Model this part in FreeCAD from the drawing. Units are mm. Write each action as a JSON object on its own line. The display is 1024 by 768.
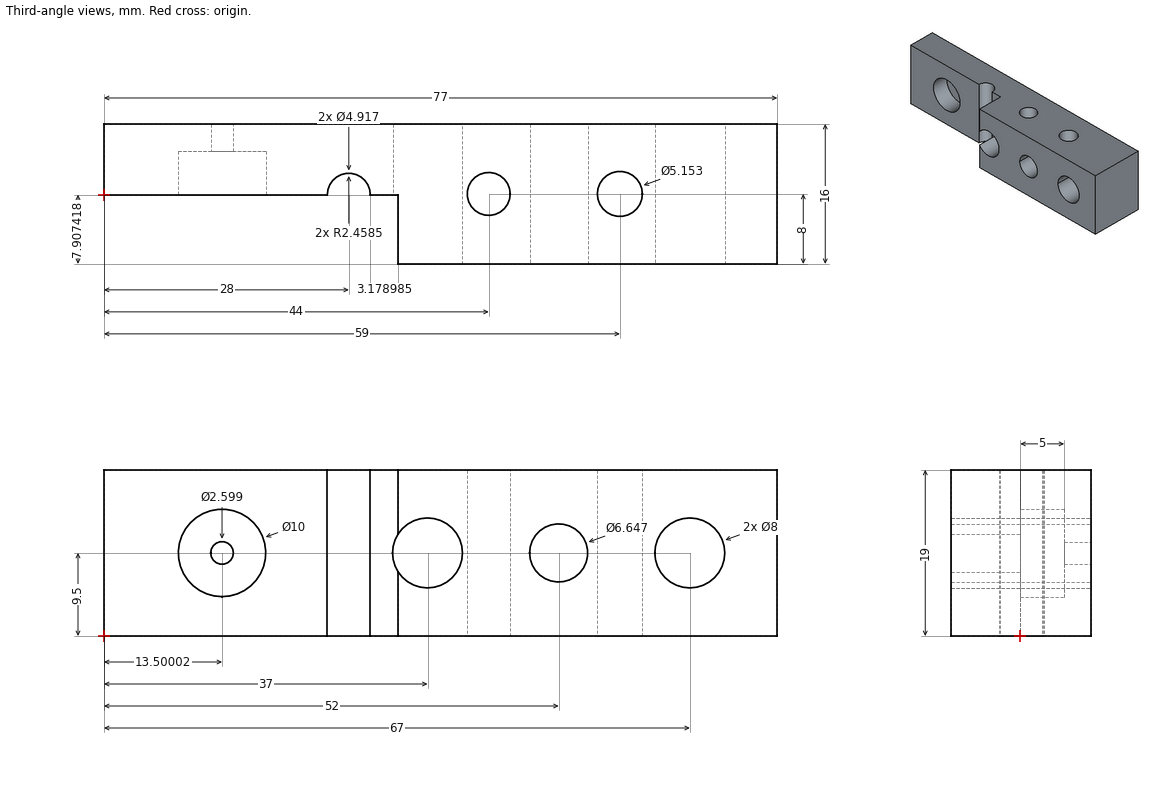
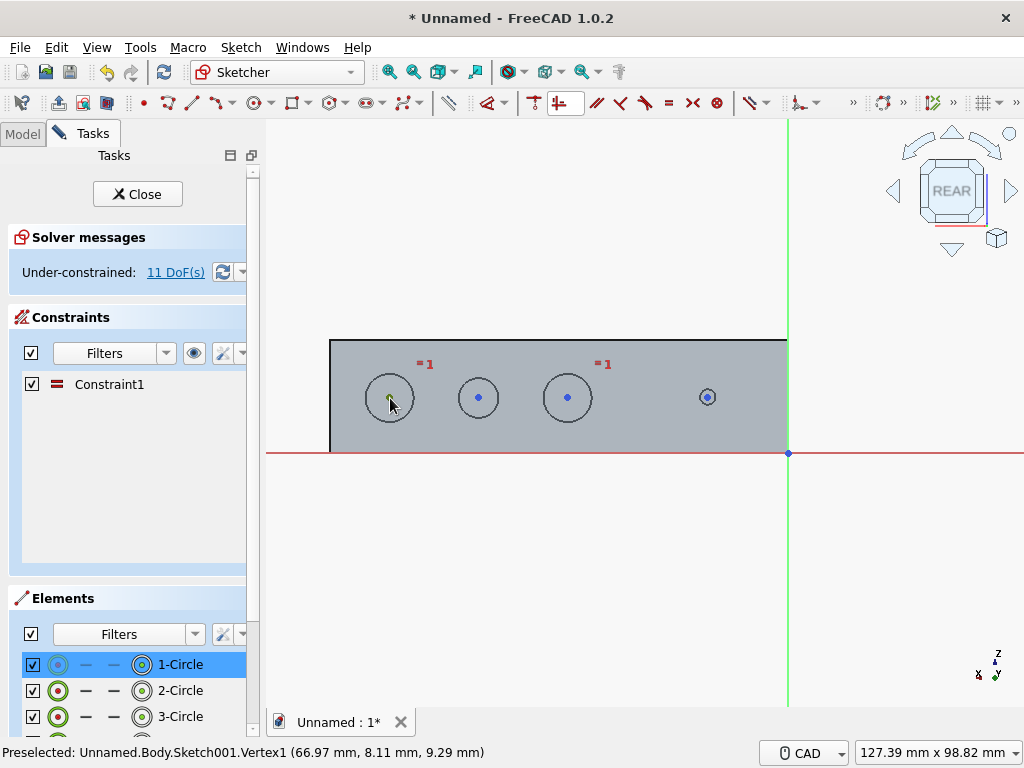
{"action": "left_click", "coordinate": [479, 398]}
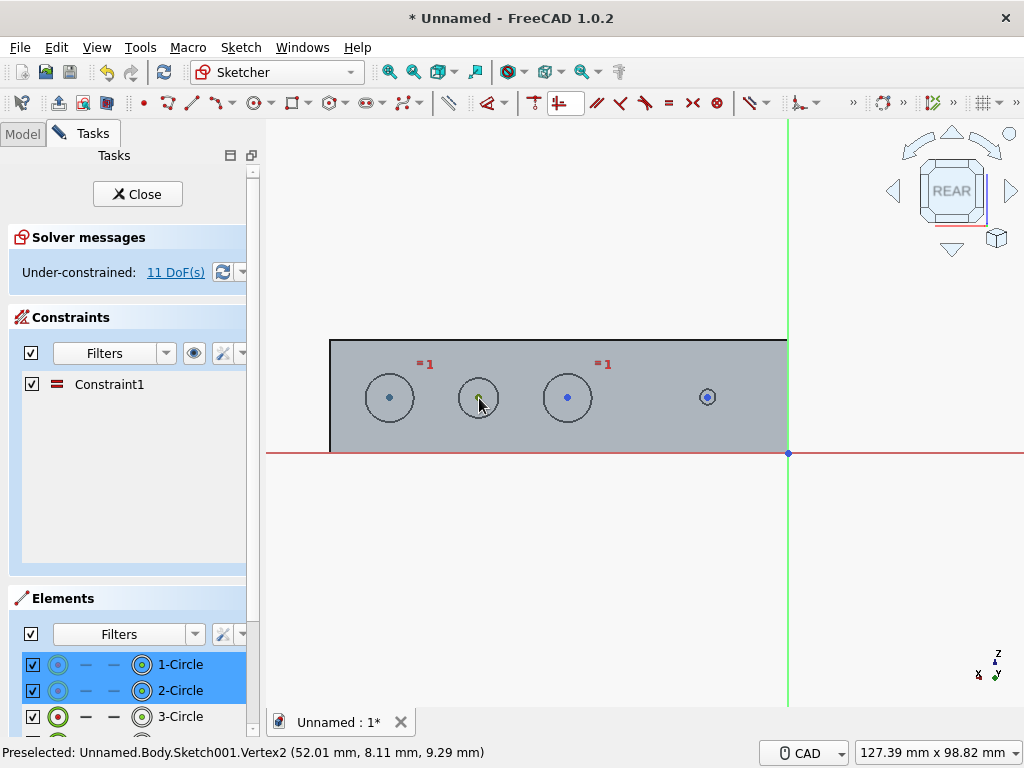
{"action": "left_click", "coordinate": [578, 104]}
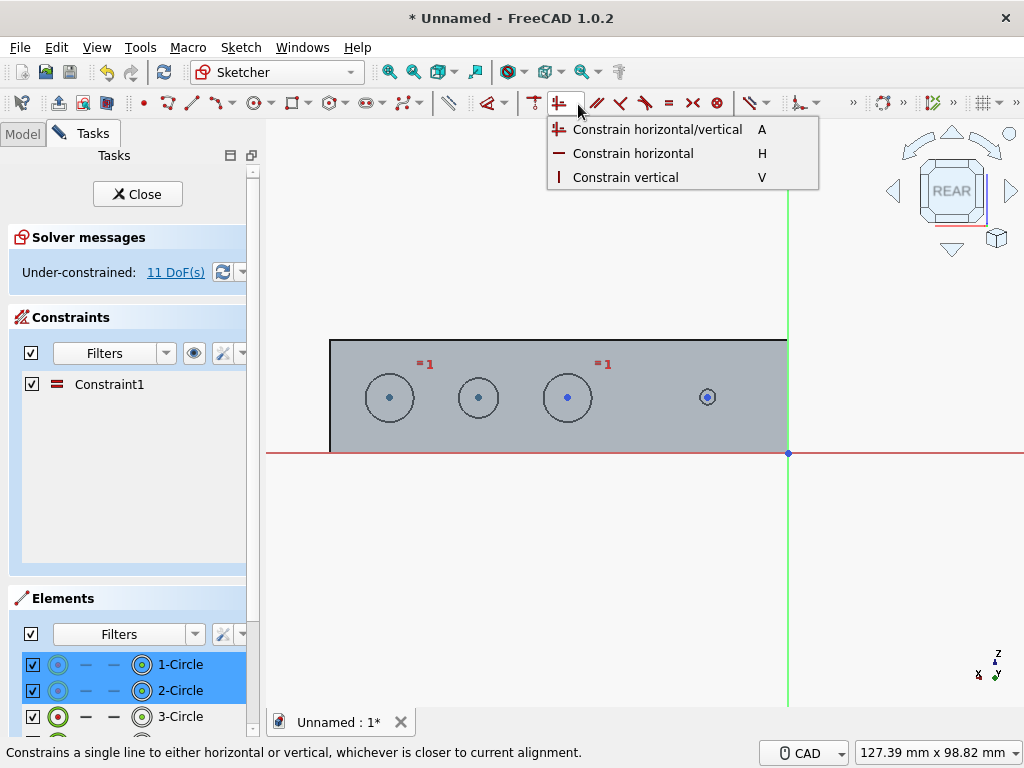
{"action": "left_click", "coordinate": [683, 153]}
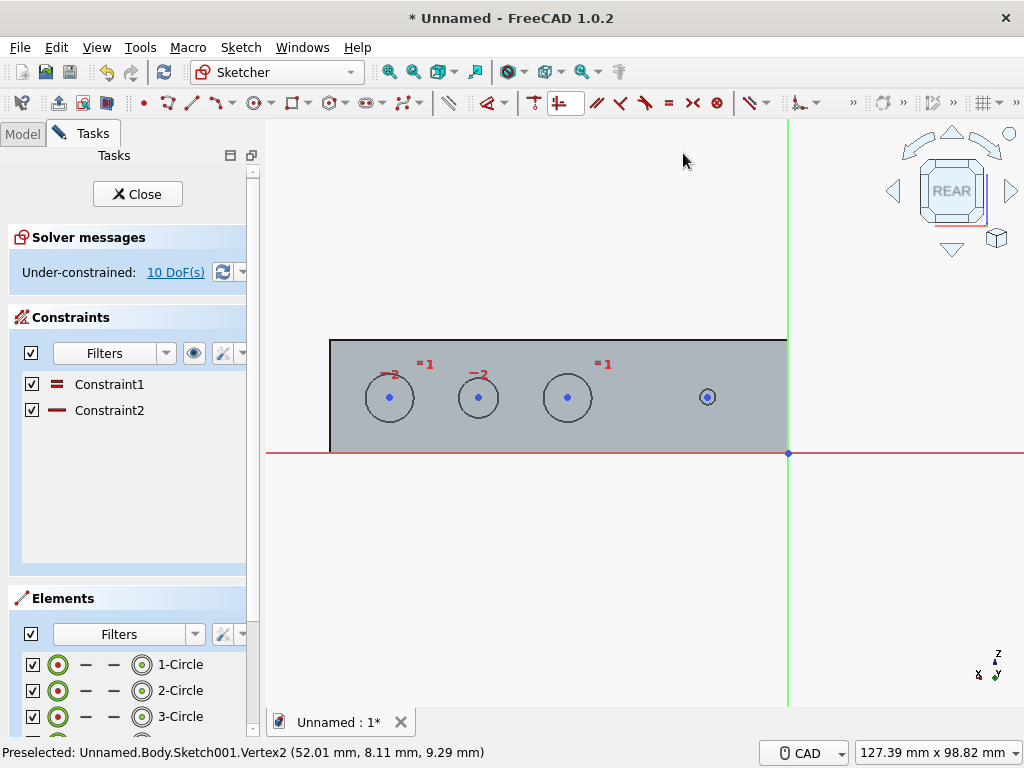
{"action": "left_click", "coordinate": [479, 398]}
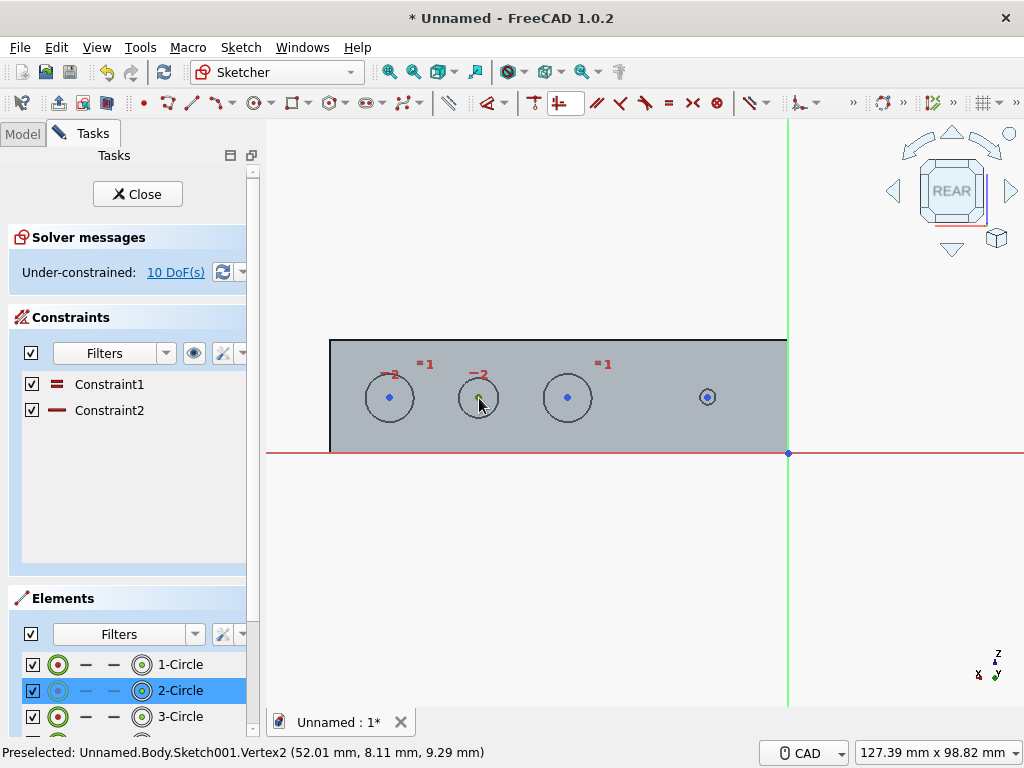
{"action": "left_click", "coordinate": [568, 398]}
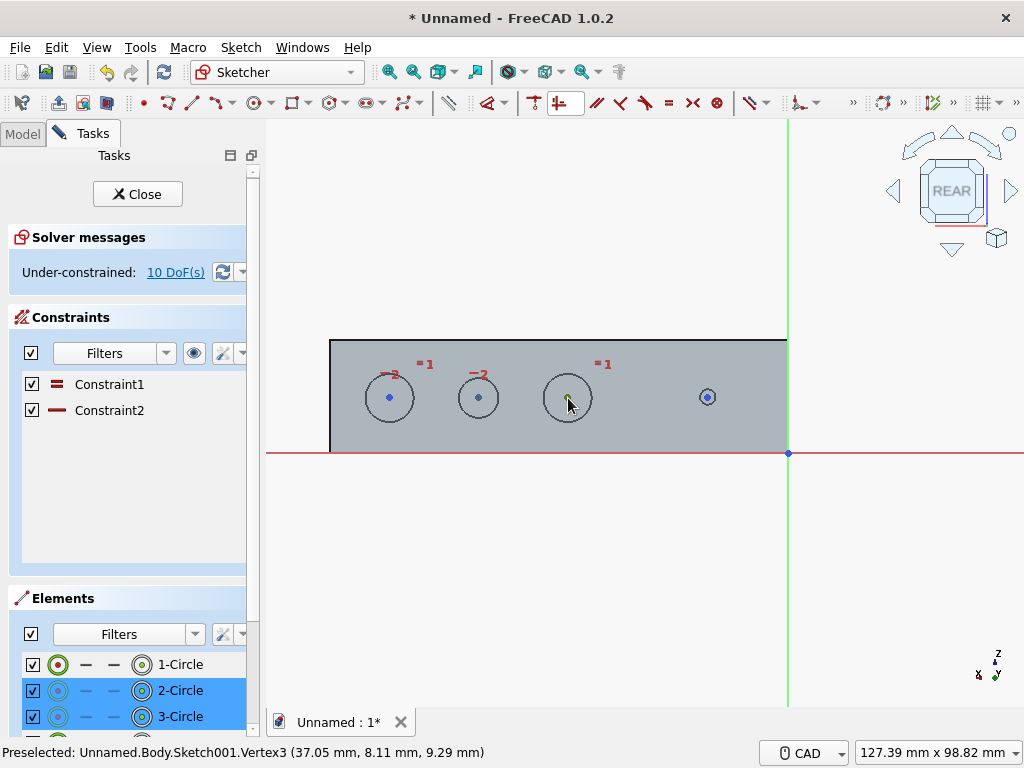
{"action": "key", "text": "h"}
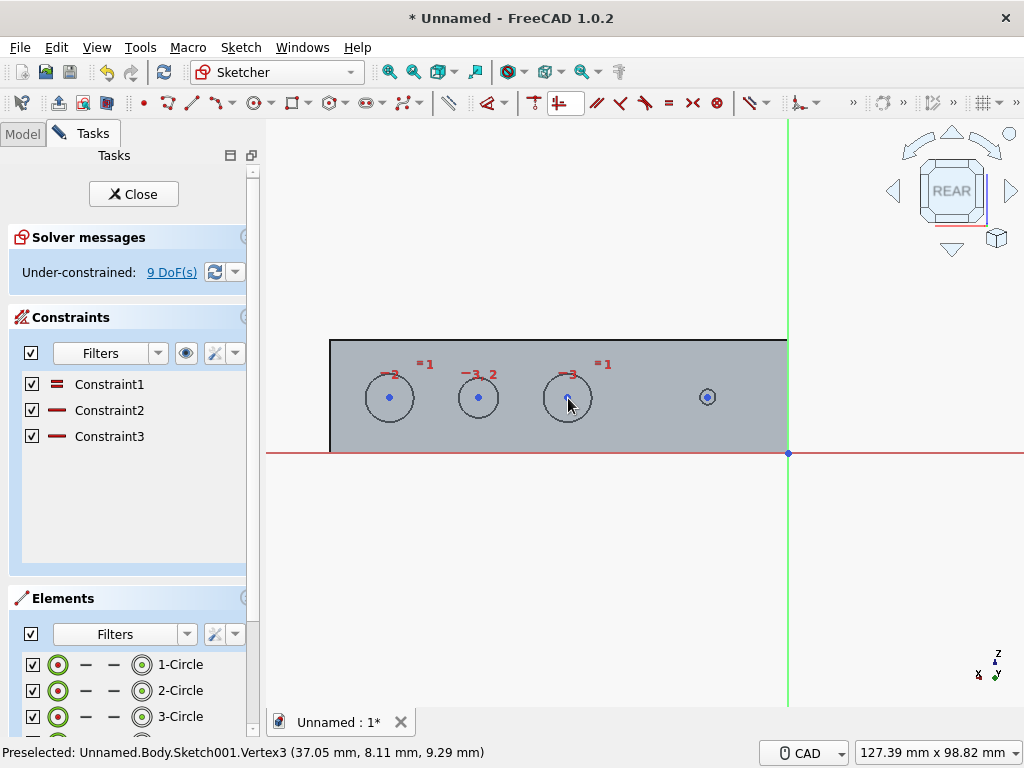
{"action": "left_click", "coordinate": [568, 398]}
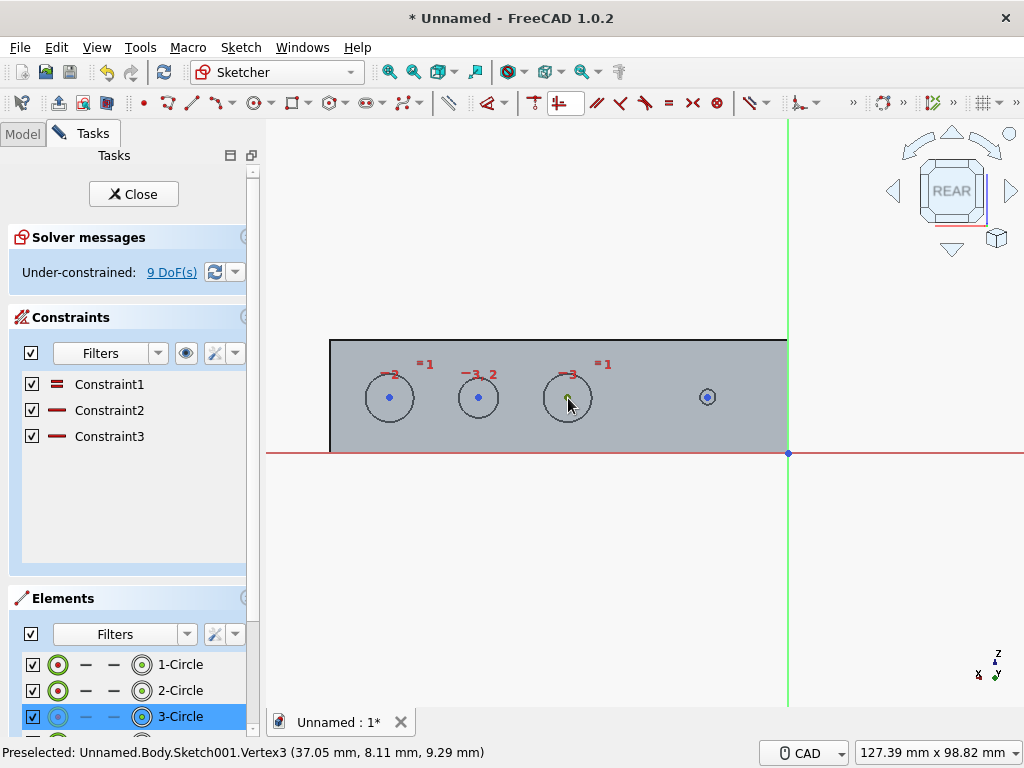
{"action": "left_click", "coordinate": [708, 397]}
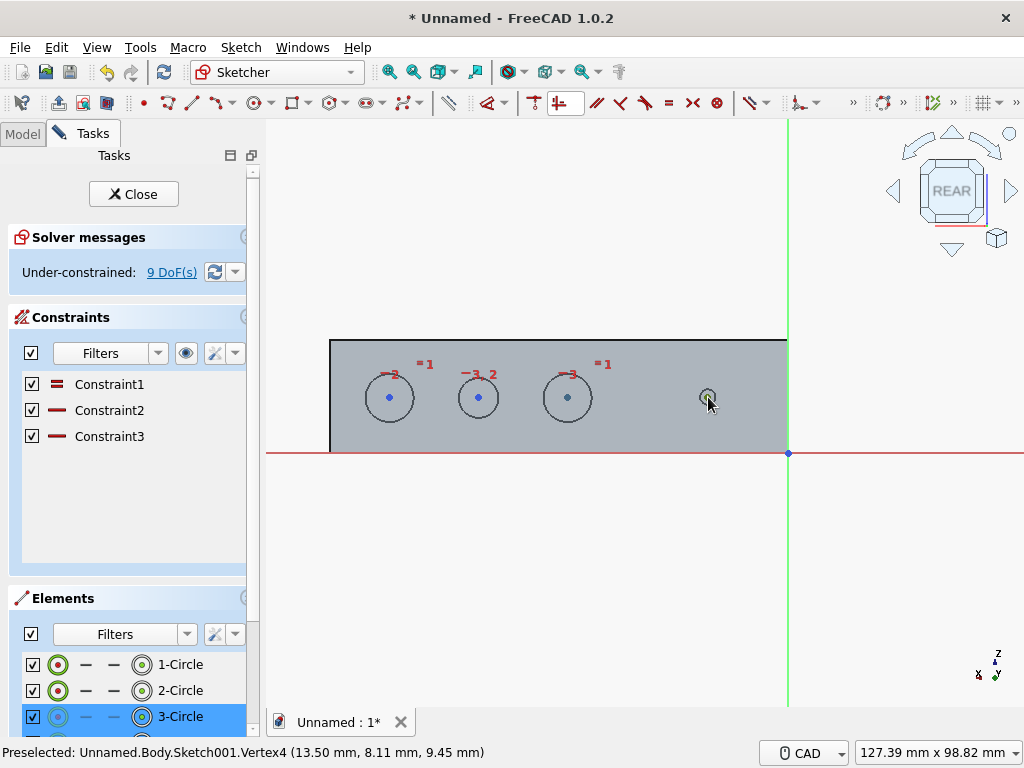
{"action": "left_click", "coordinate": [578, 104]}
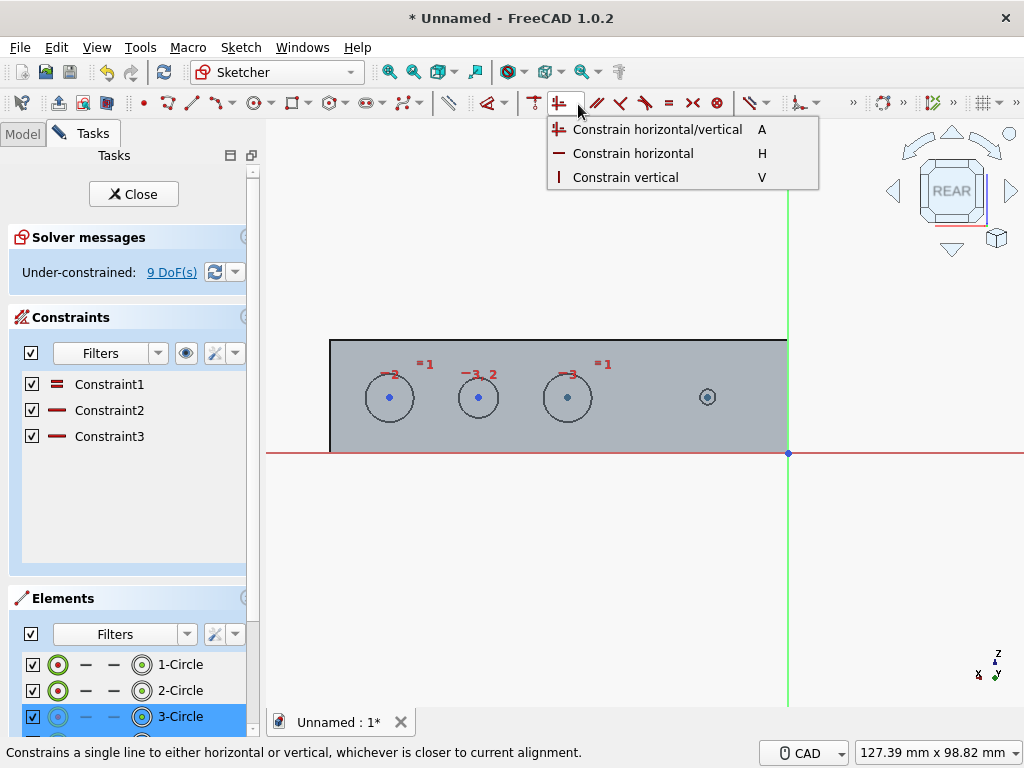
{"action": "left_click", "coordinate": [683, 153]}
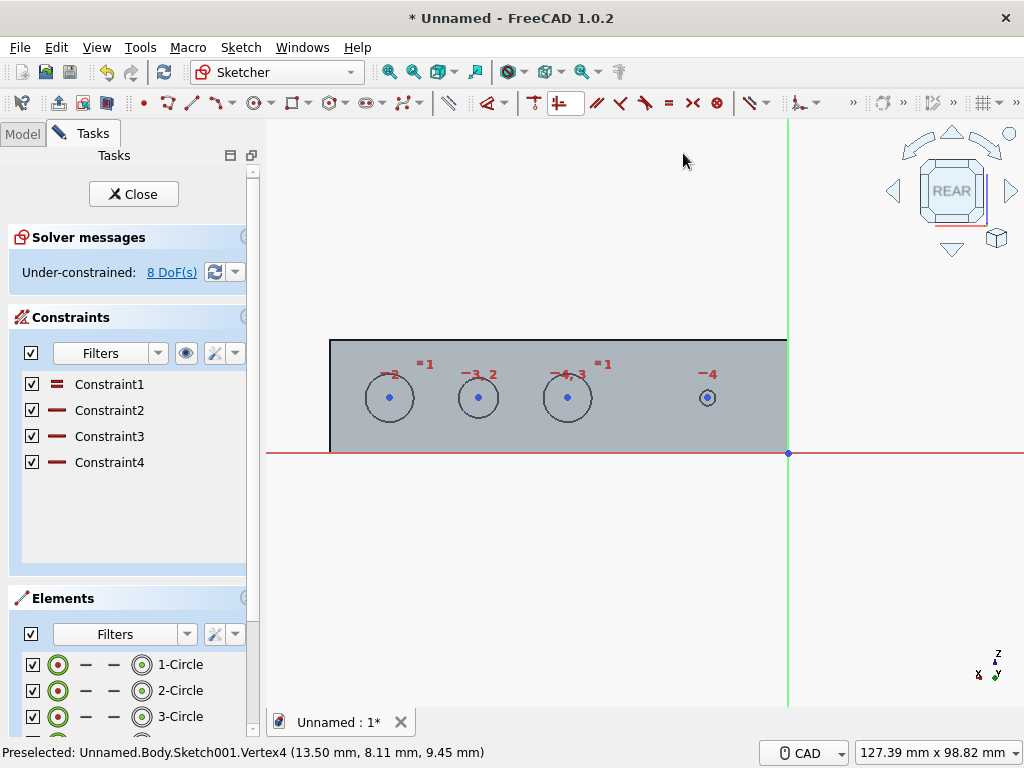
{"action": "left_click", "coordinate": [488, 104]}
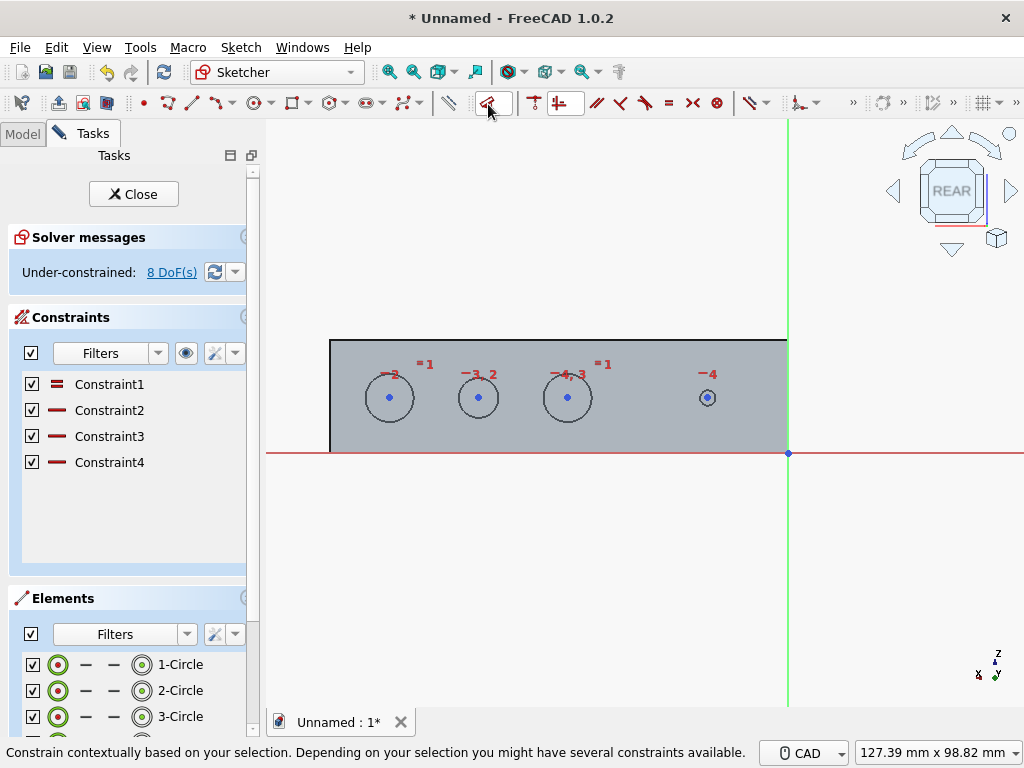
{"action": "left_click", "coordinate": [407, 381]}
{"action": "left_click", "coordinate": [430, 359]}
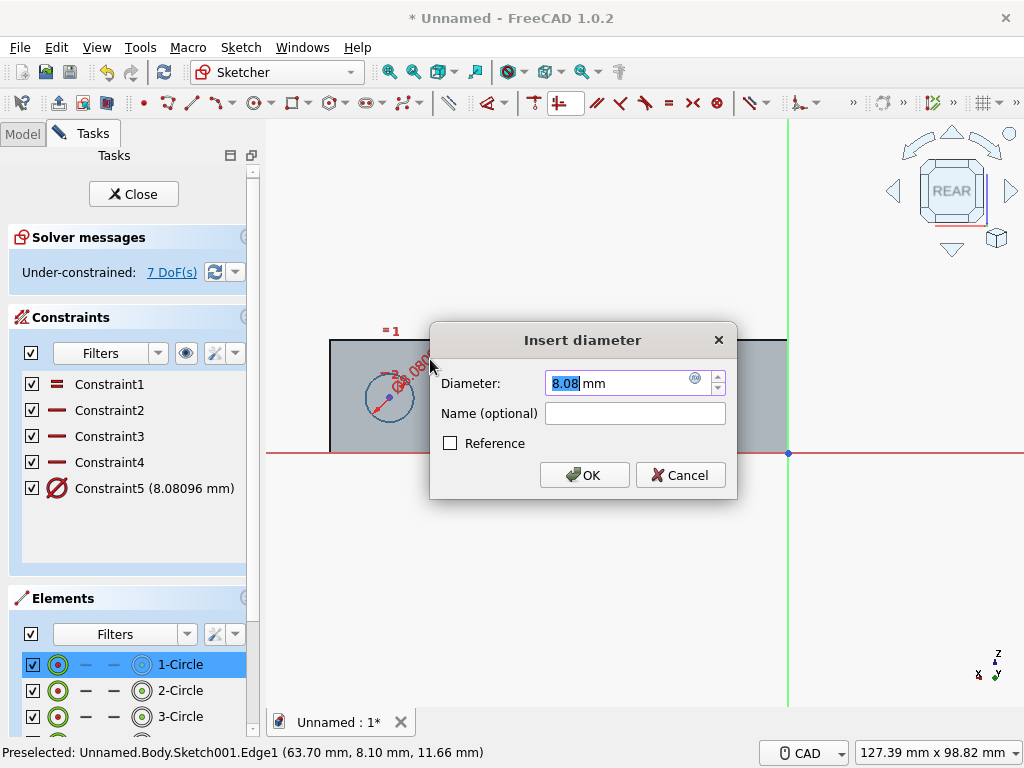
{"action": "type", "text": "8"}
{"action": "key", "text": "Return"}